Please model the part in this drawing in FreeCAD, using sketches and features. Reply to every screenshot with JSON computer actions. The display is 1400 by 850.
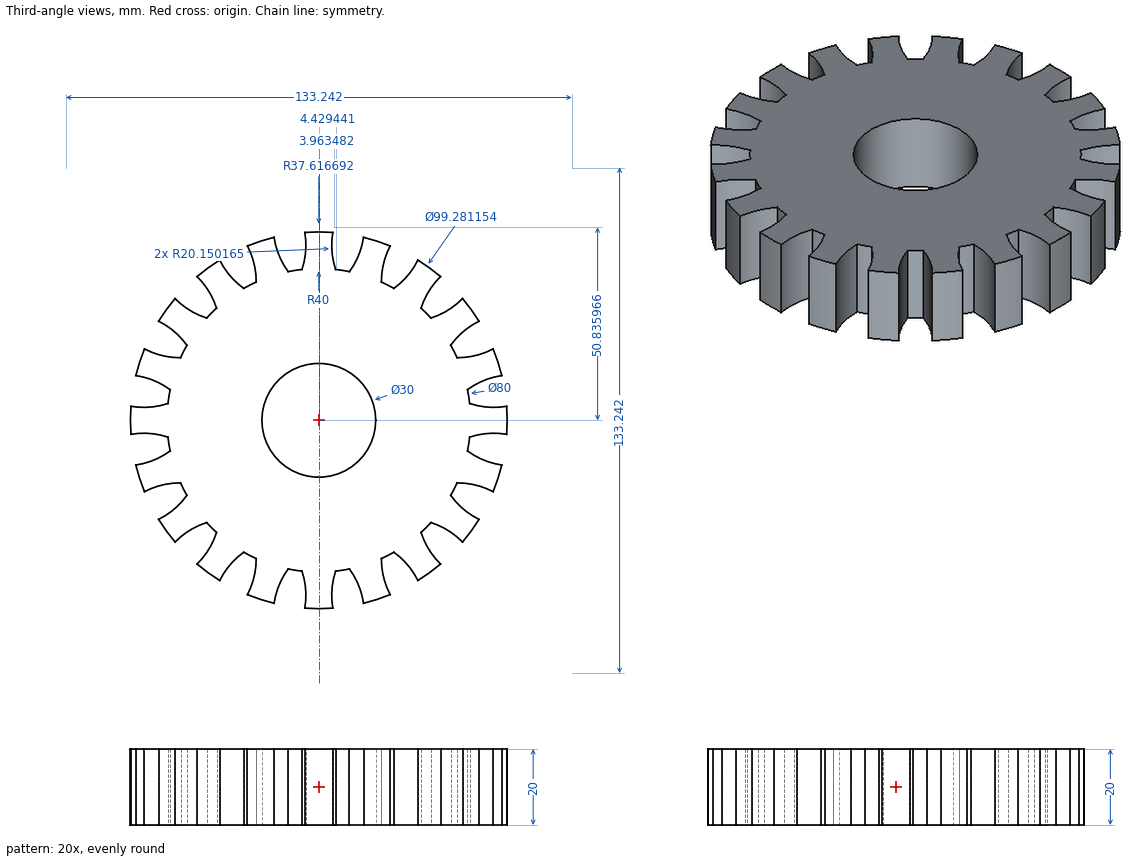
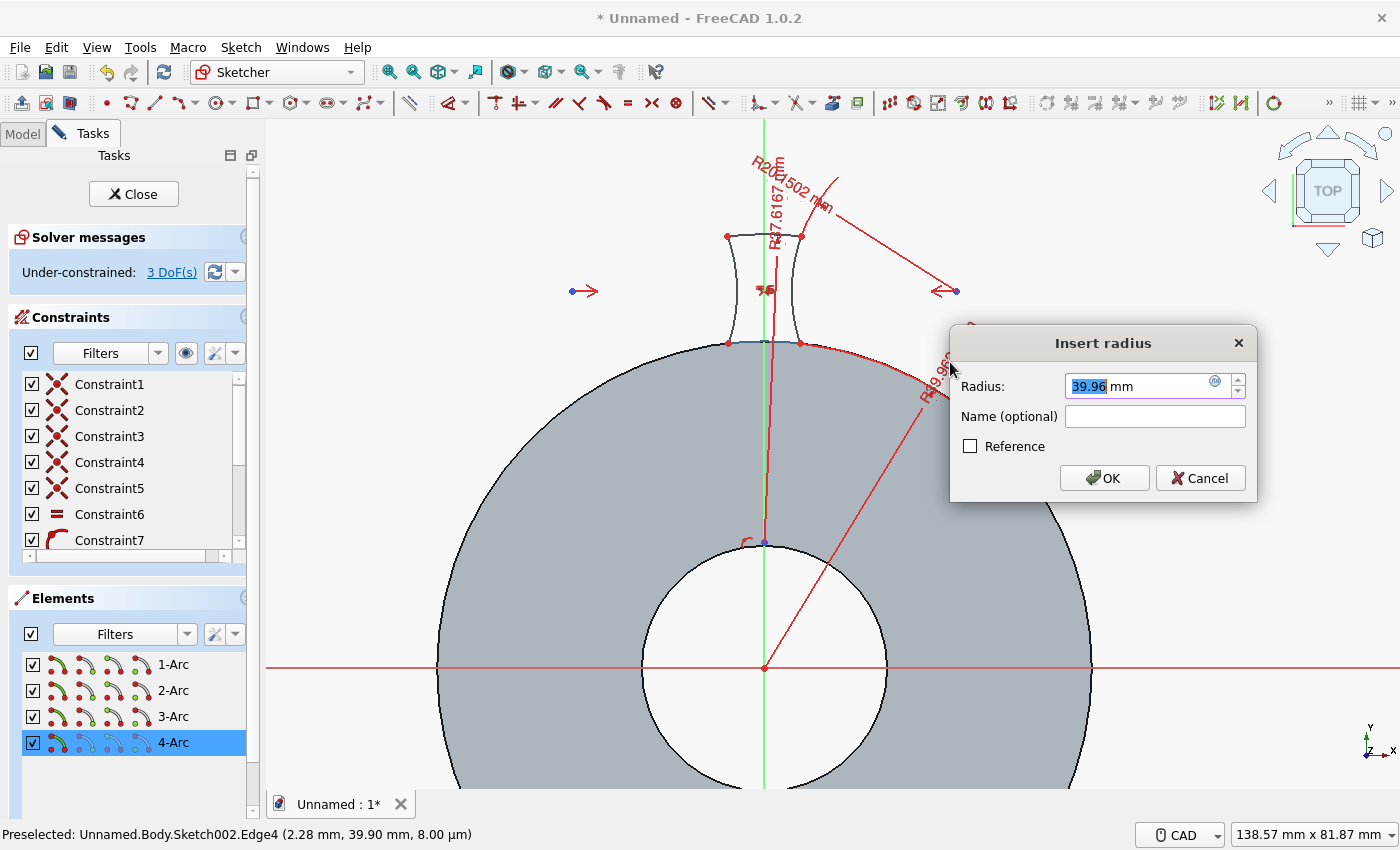
{"action": "type", "text": "40"}
{"action": "key", "text": "Return"}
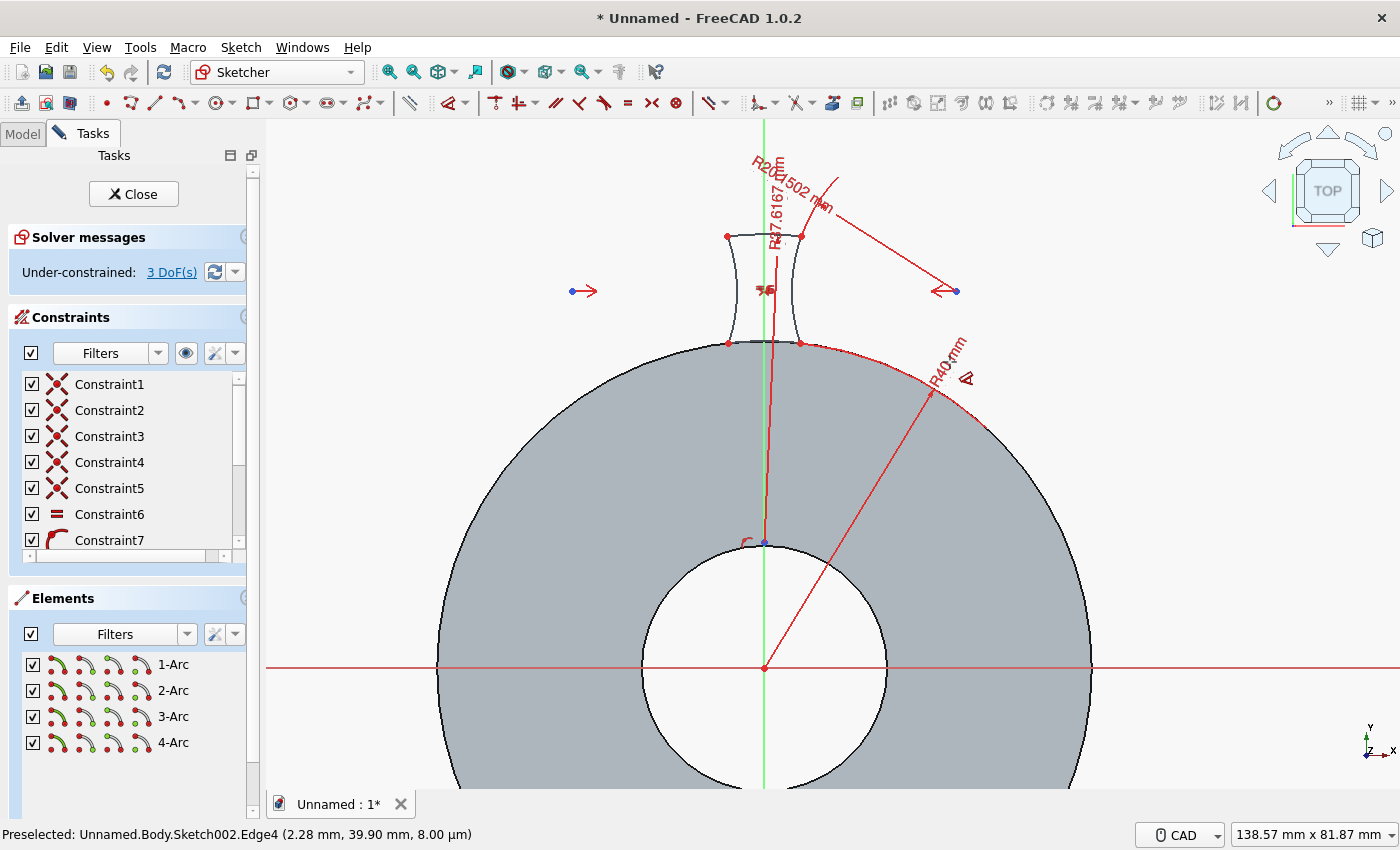
{"action": "scroll", "coordinate": [801, 237], "scroll_direction": "up", "scroll_amount": 2}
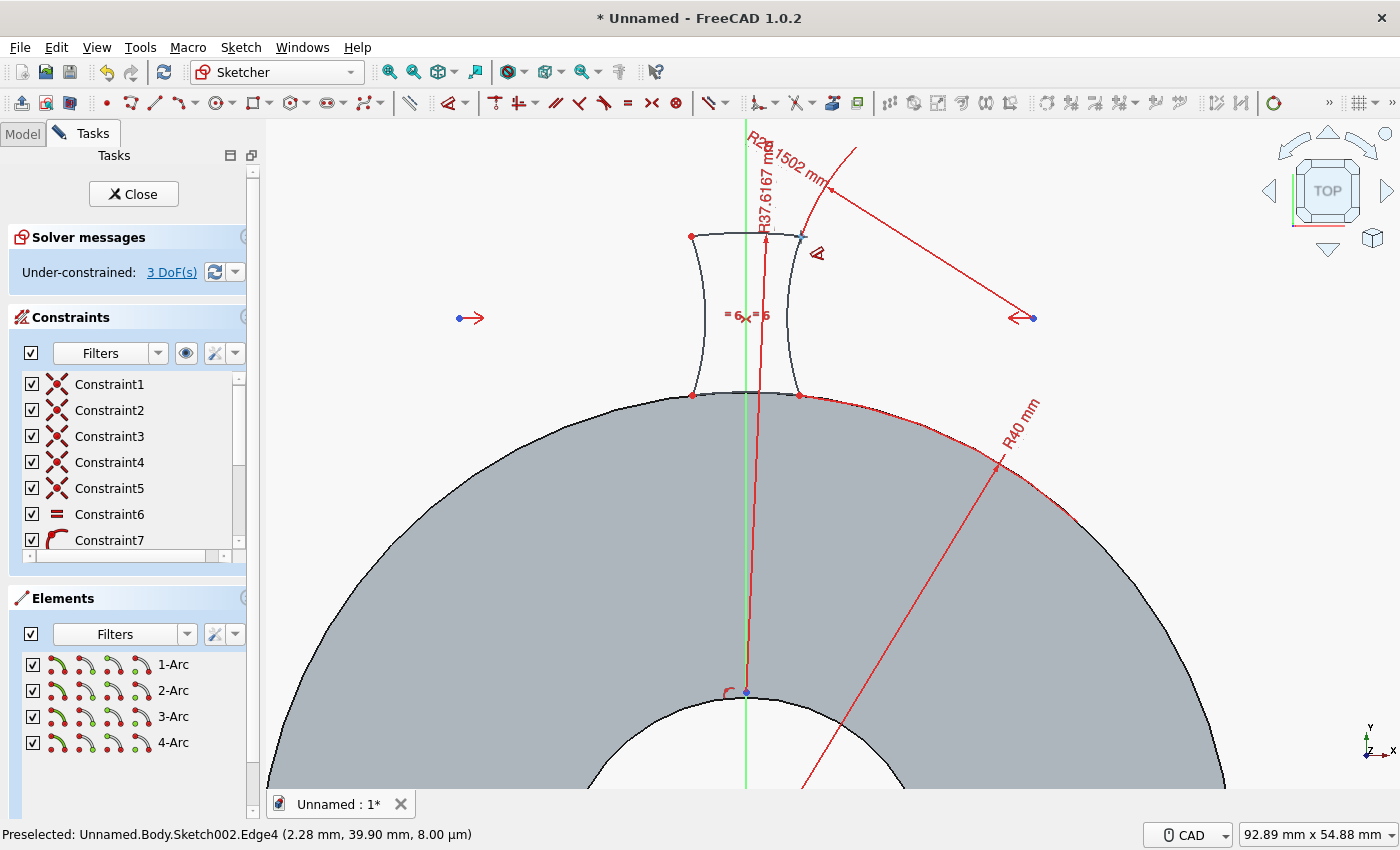
{"action": "left_click", "coordinate": [801, 236]}
{"action": "left_click", "coordinate": [774, 178]}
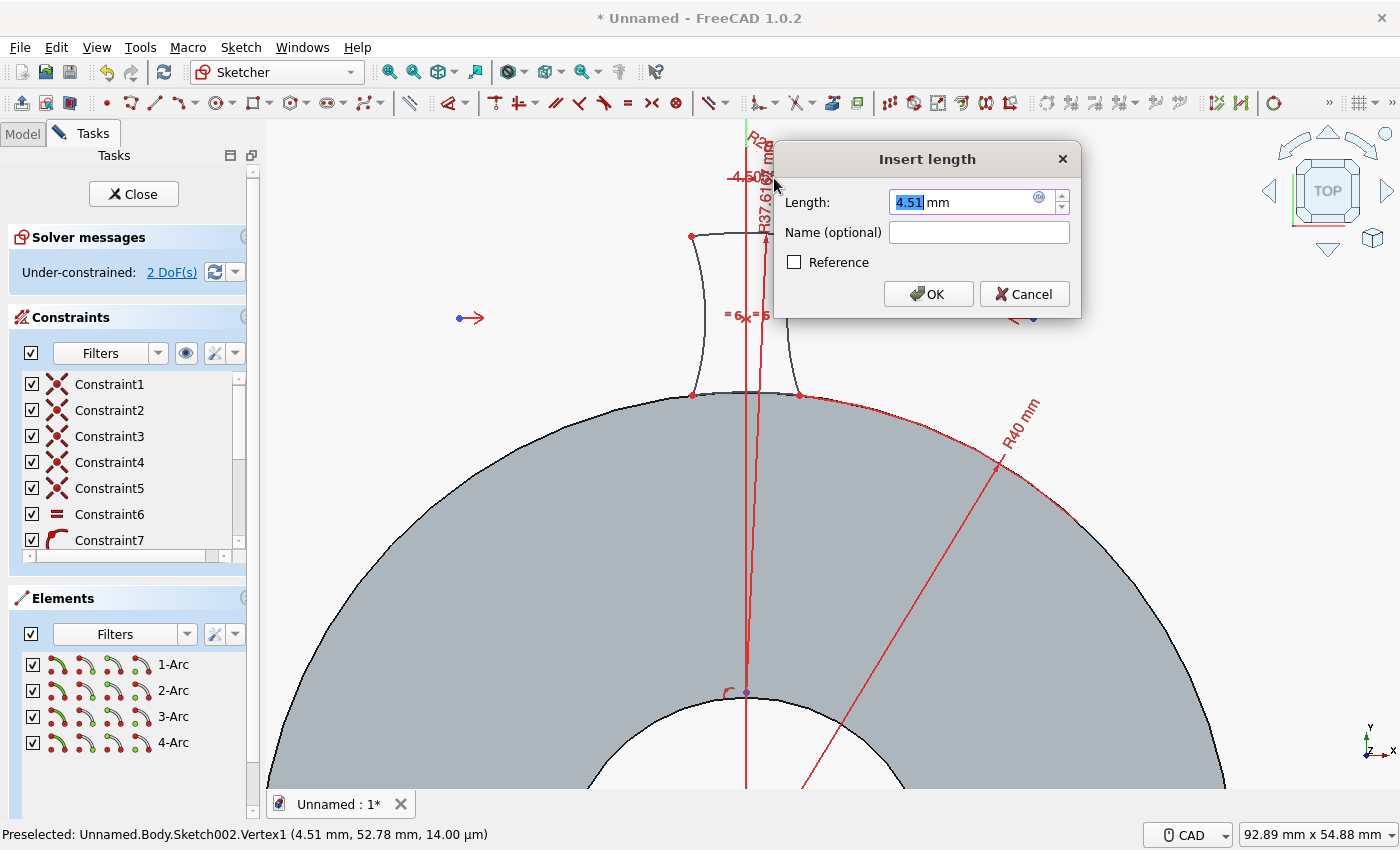
{"action": "type", "text": "3.963482"}
{"action": "key", "text": "Return"}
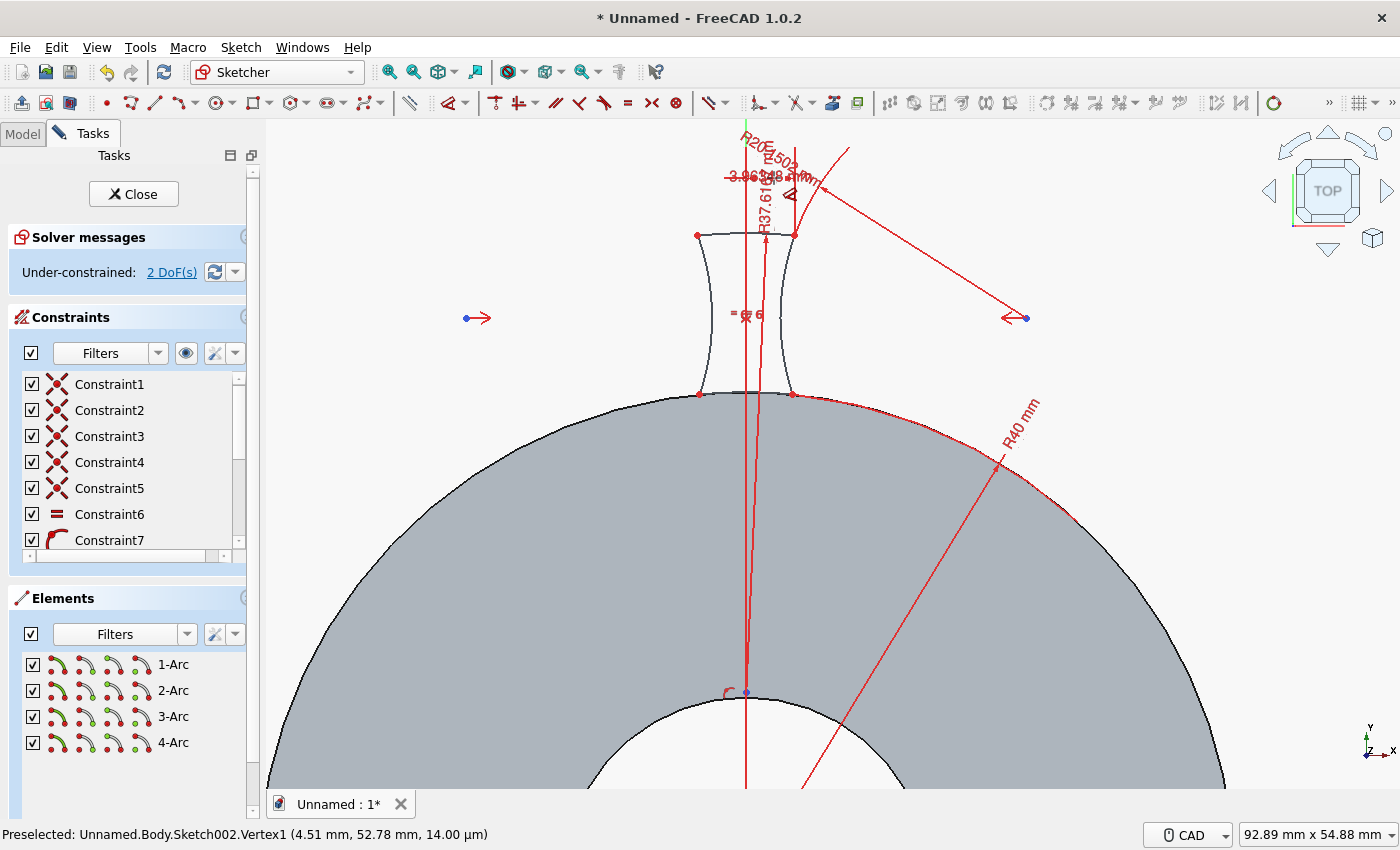
{"action": "left_click", "coordinate": [793, 395]}
{"action": "left_click", "coordinate": [769, 361]}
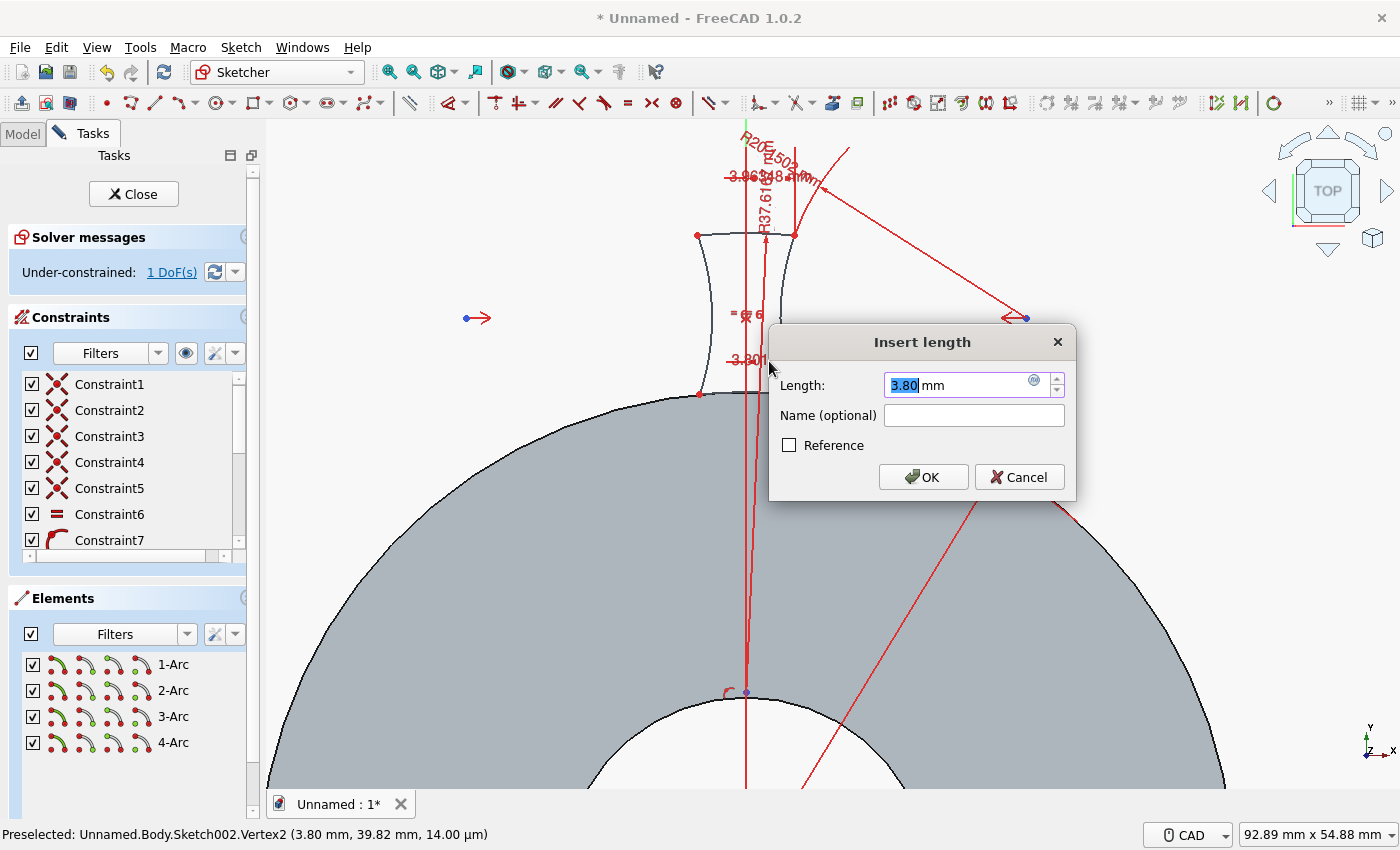
{"action": "type", "text": "4.429441"}
{"action": "key", "text": "Return"}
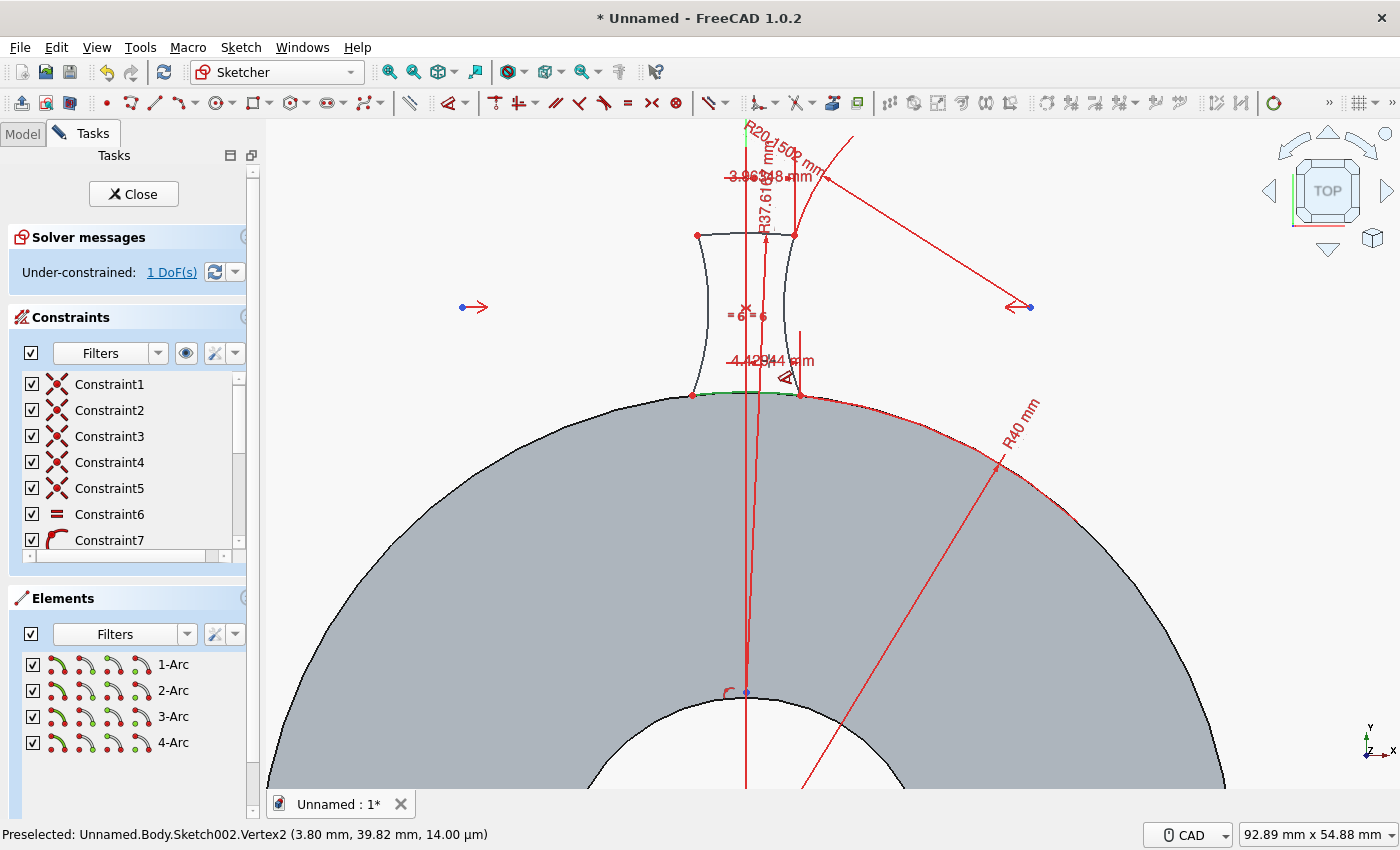
{"action": "left_click", "coordinate": [795, 236]}
{"action": "left_click", "coordinate": [829, 498]}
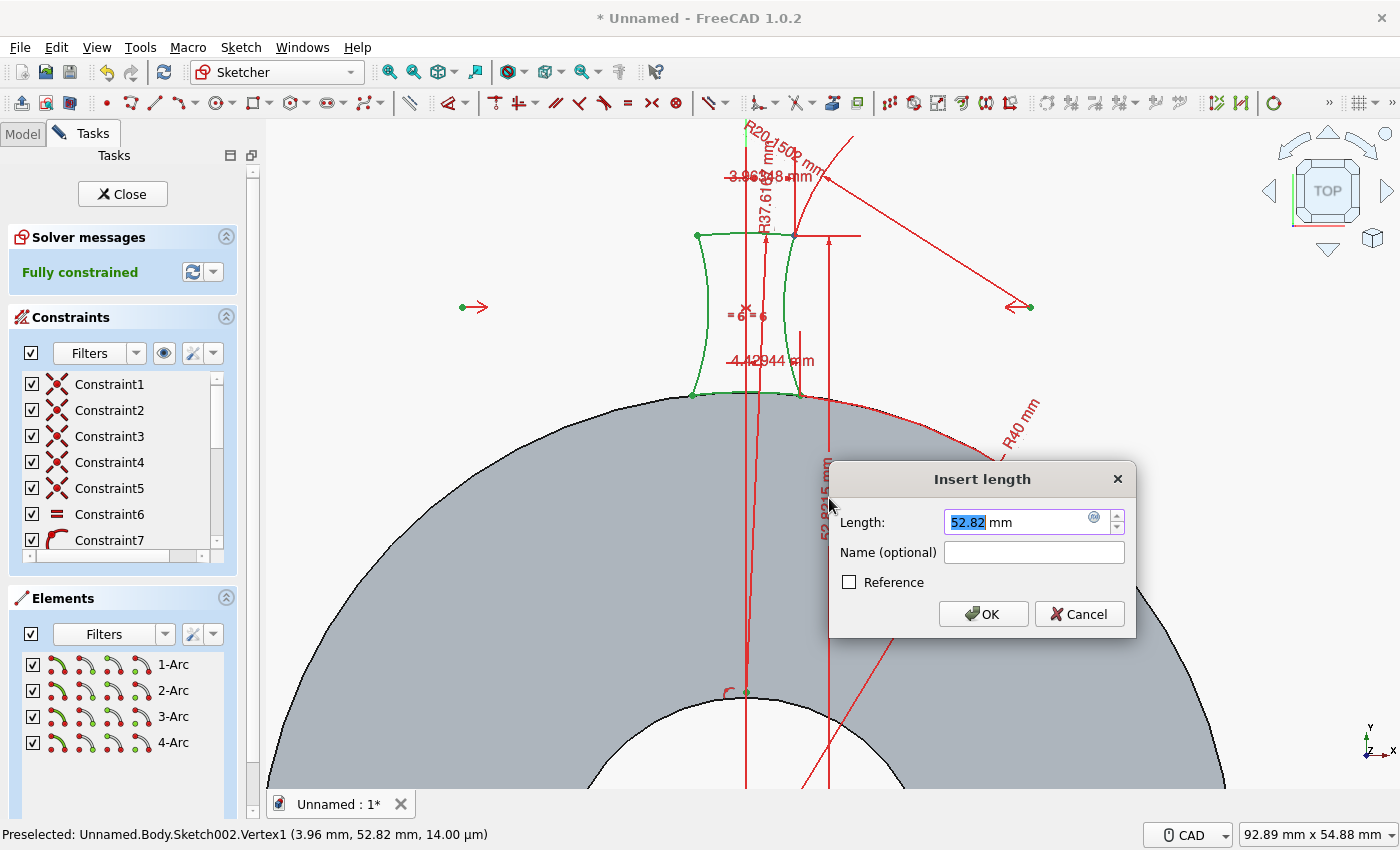
{"action": "type", "text": "50.835966"}
{"action": "key", "text": "Return"}
{"action": "key", "text": "Escape"}